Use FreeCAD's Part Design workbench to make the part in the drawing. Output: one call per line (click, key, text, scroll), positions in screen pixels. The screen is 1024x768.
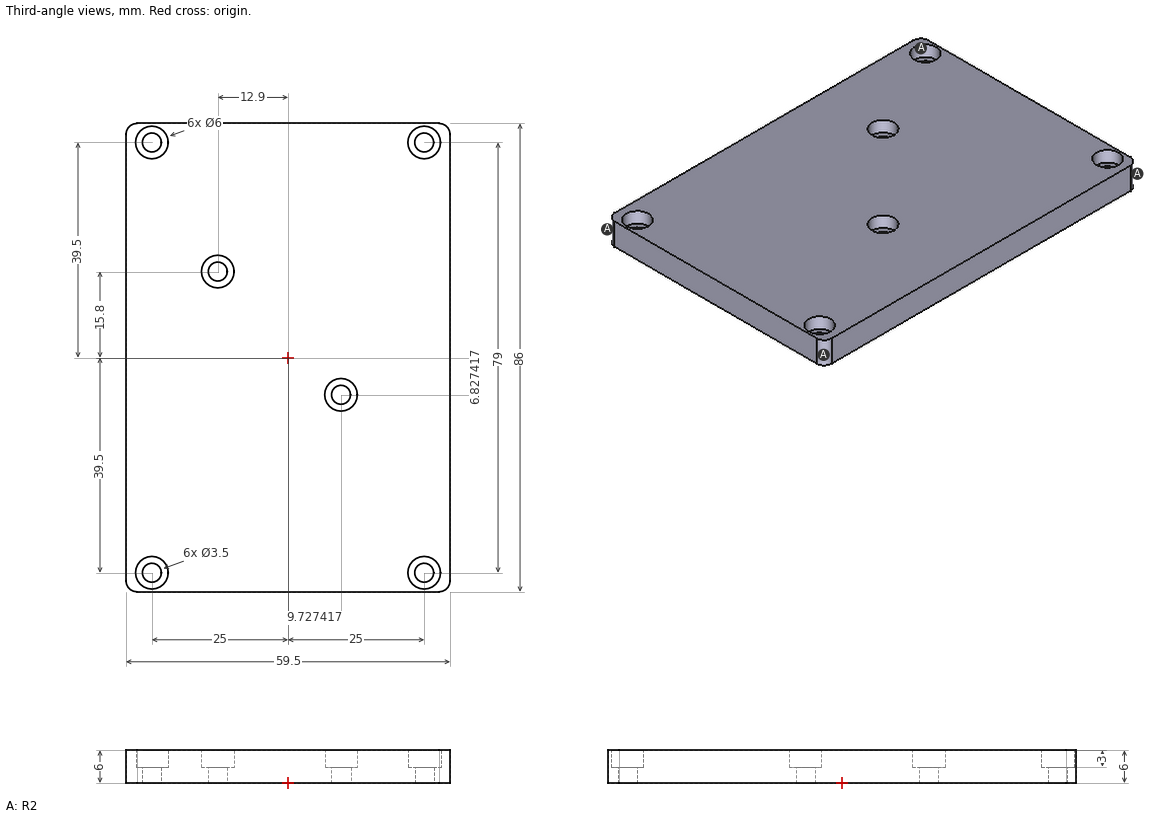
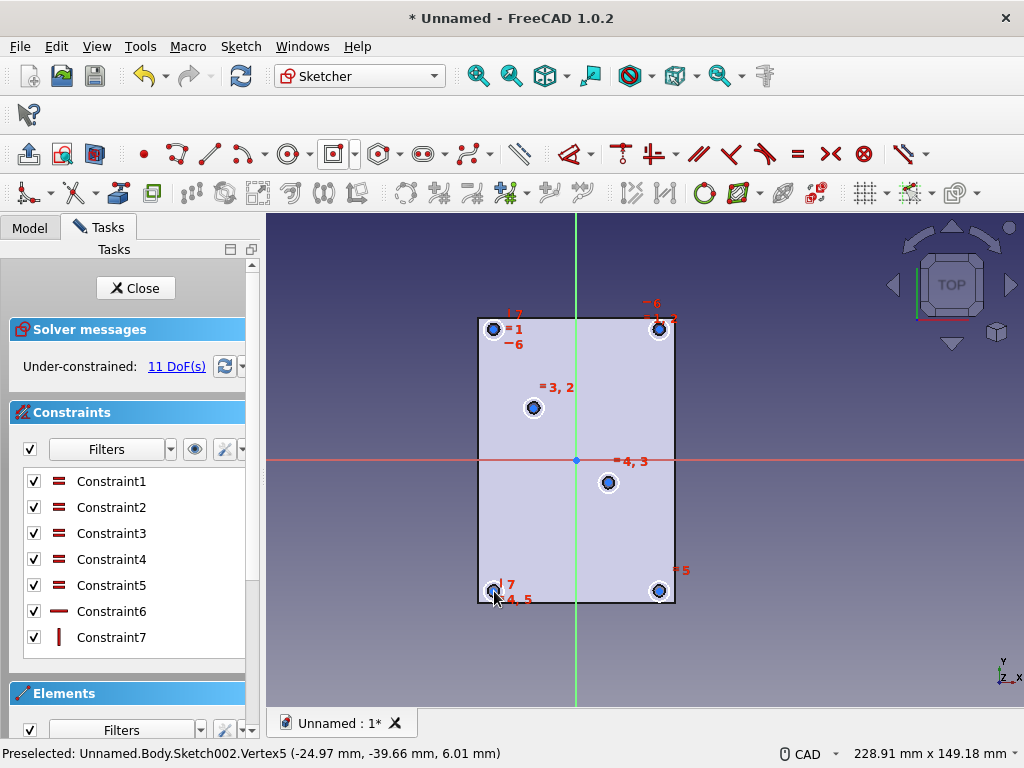
click(659, 330)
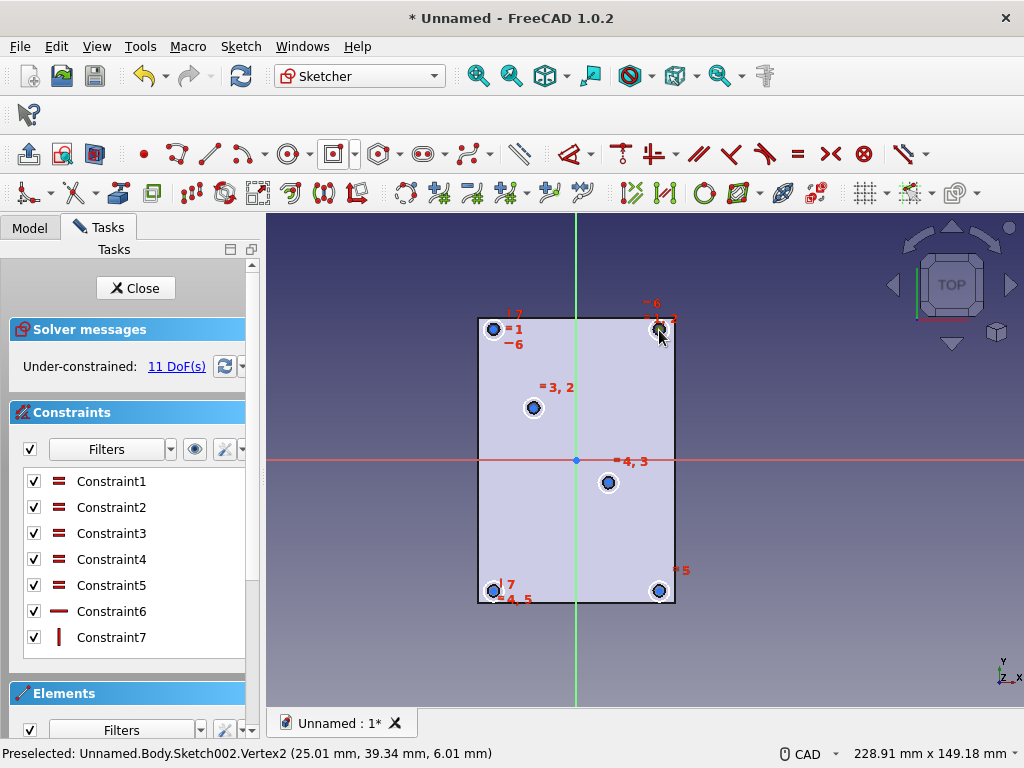
click(659, 591)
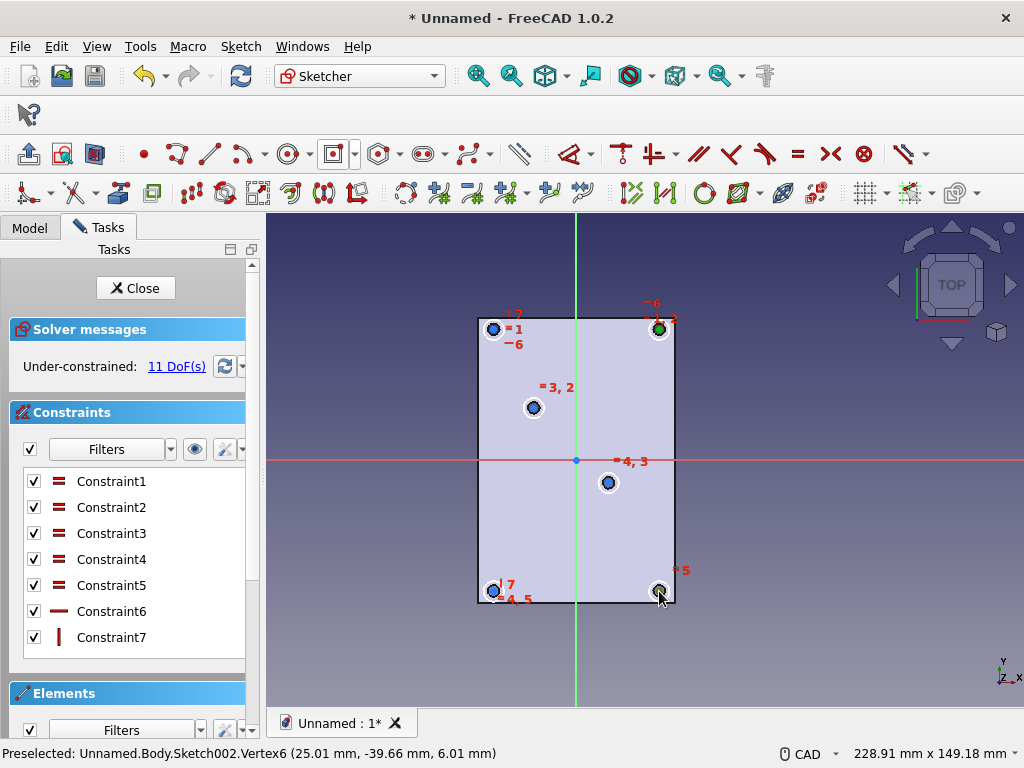
key(v)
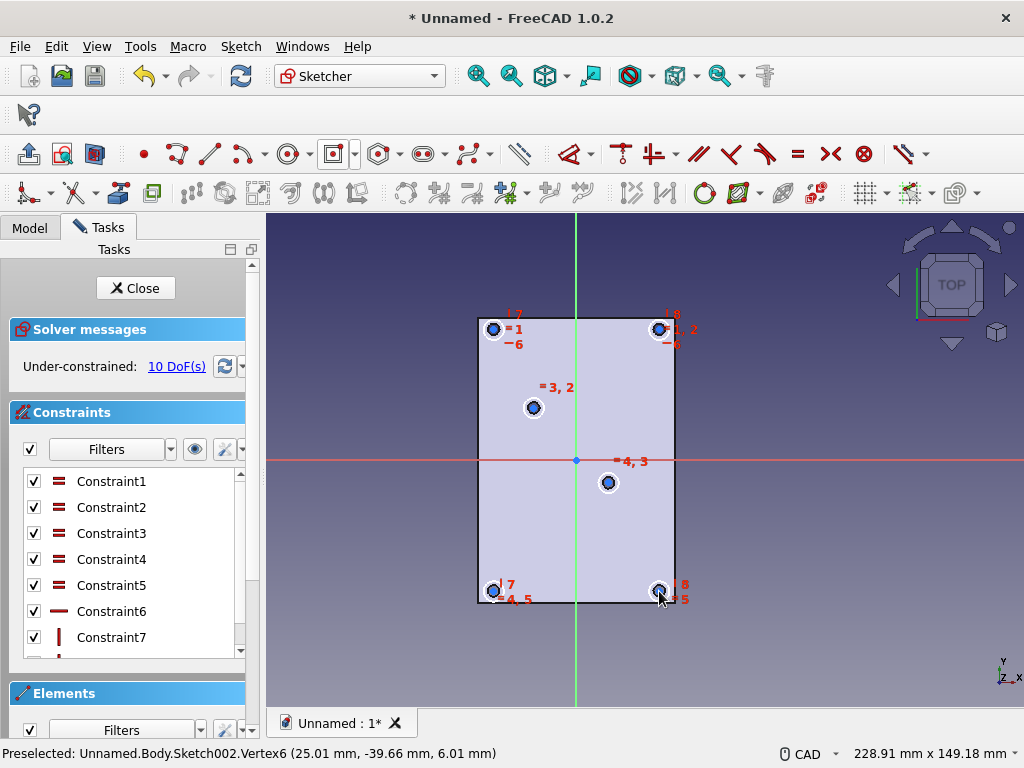
click(494, 591)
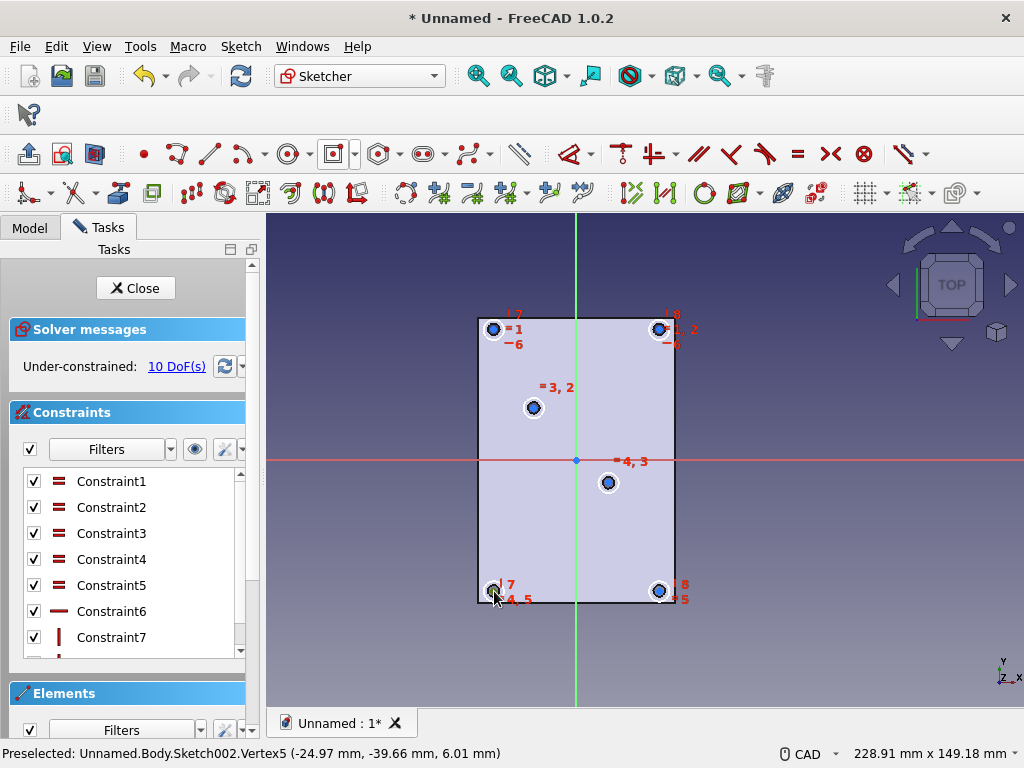
click(659, 591)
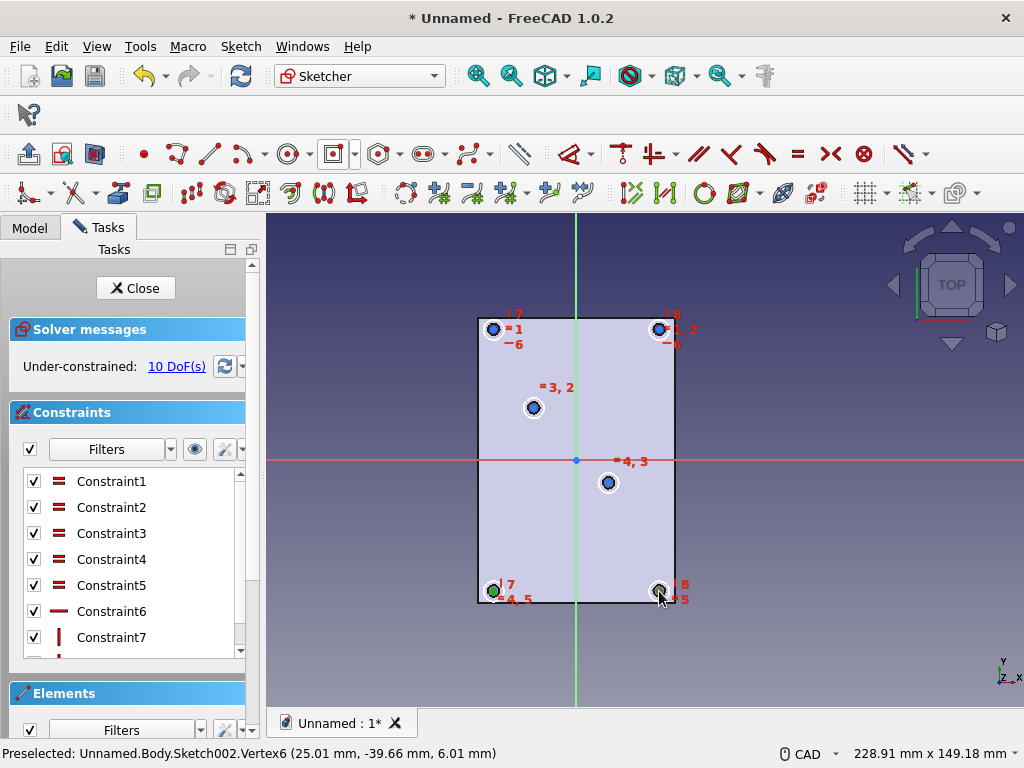
key(h)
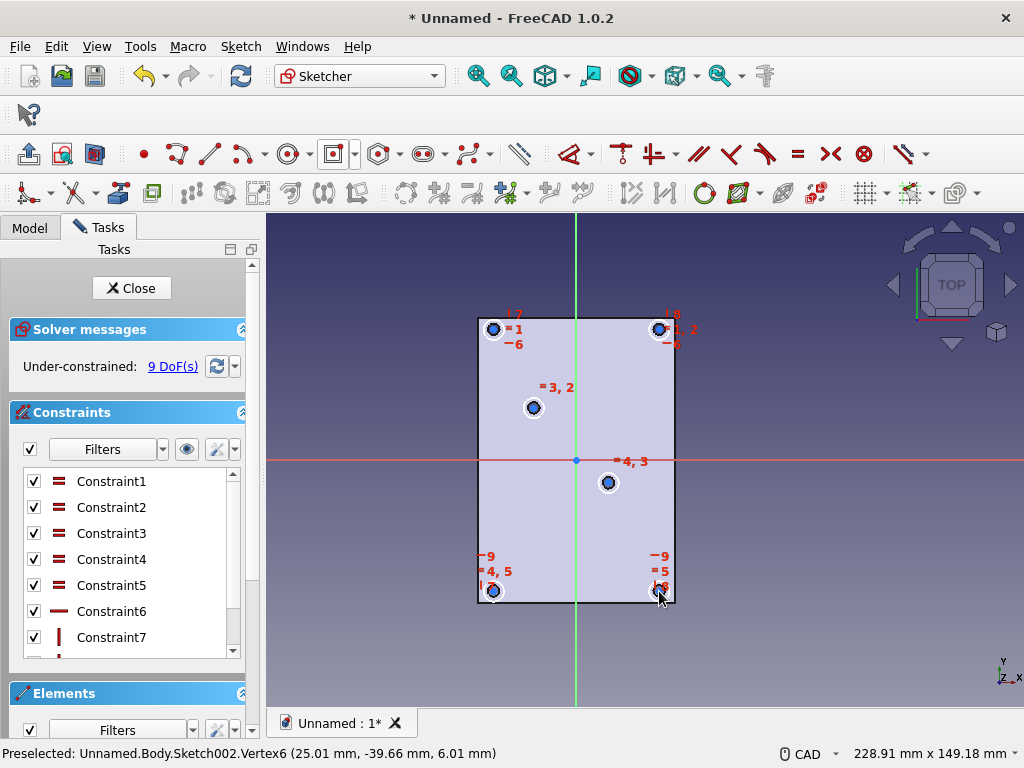
click(568, 154)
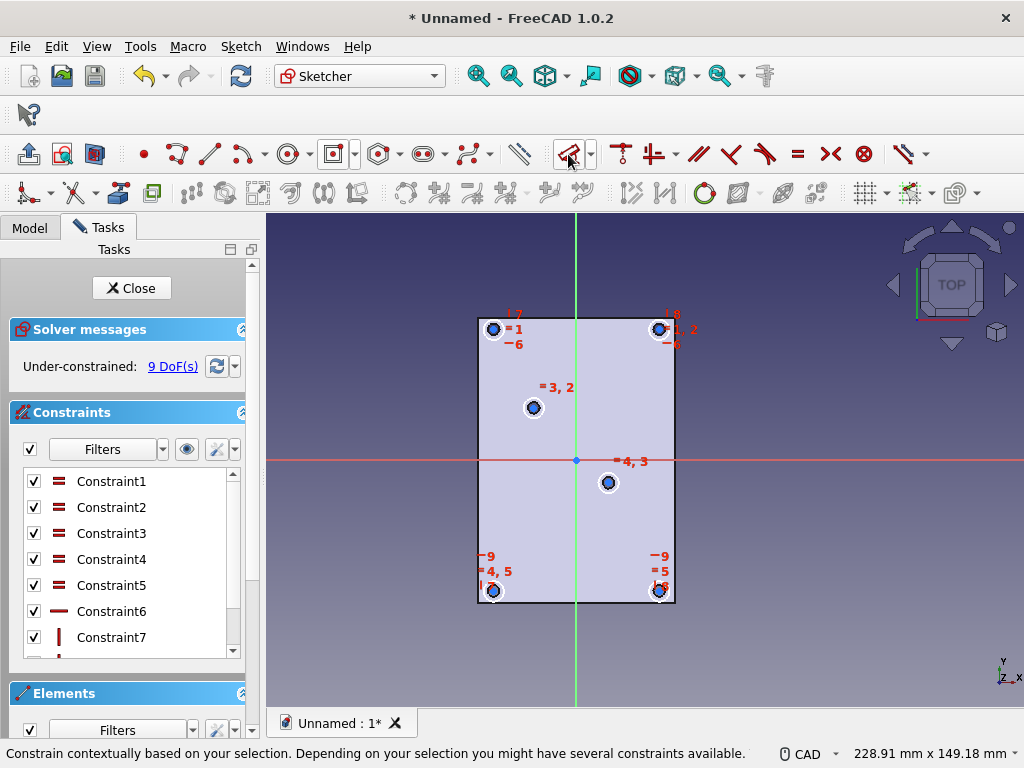
scroll(501, 323, up, 4)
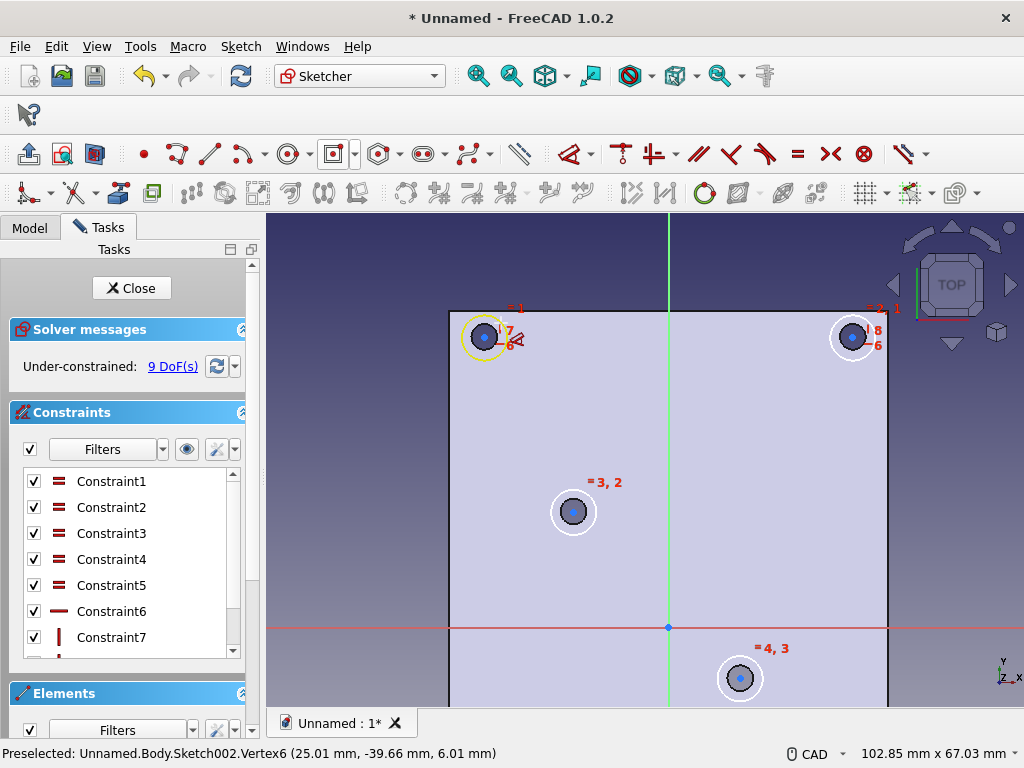
click(501, 322)
click(524, 300)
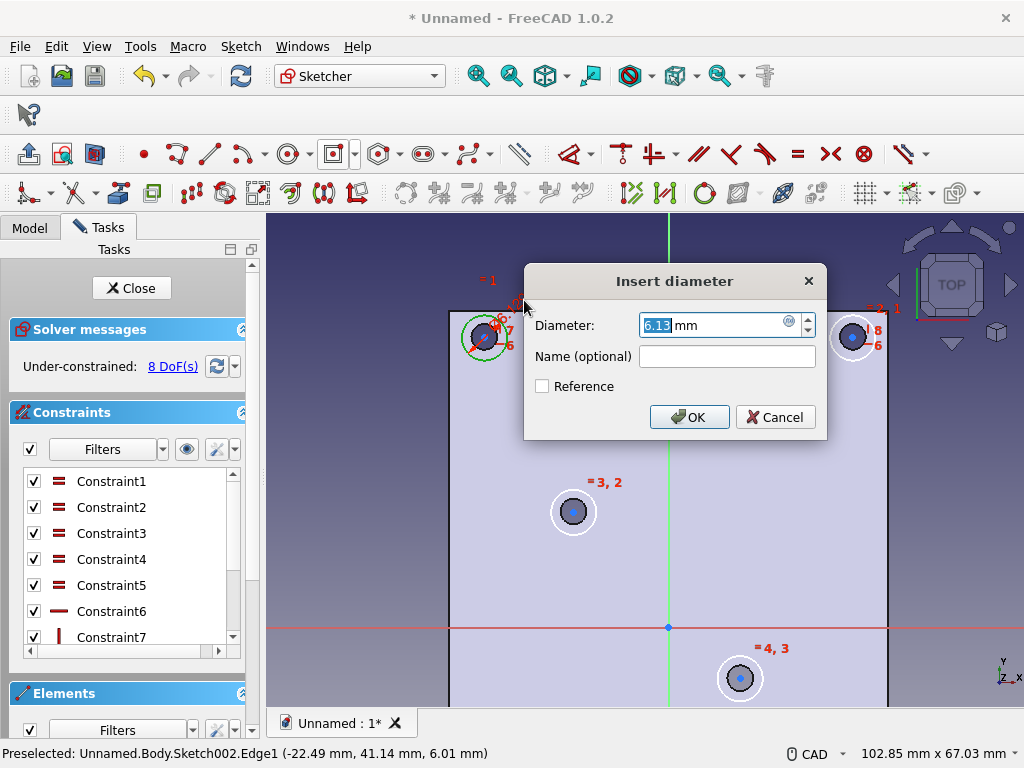
text(6)
key(Return)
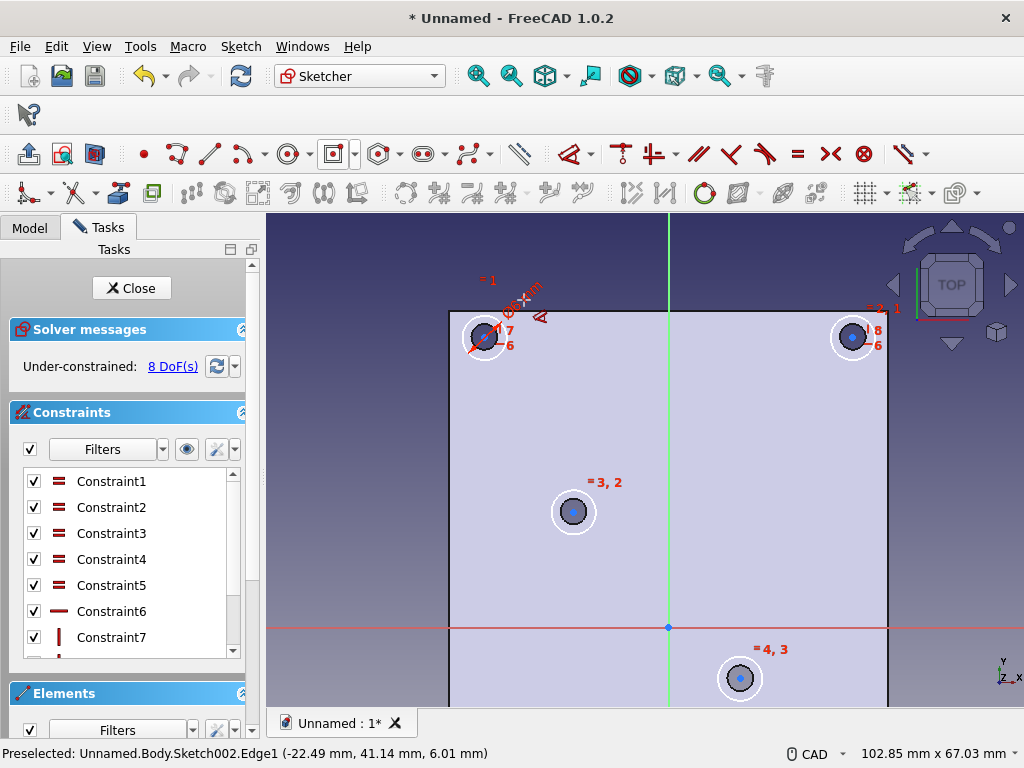
click(485, 338)
click(619, 304)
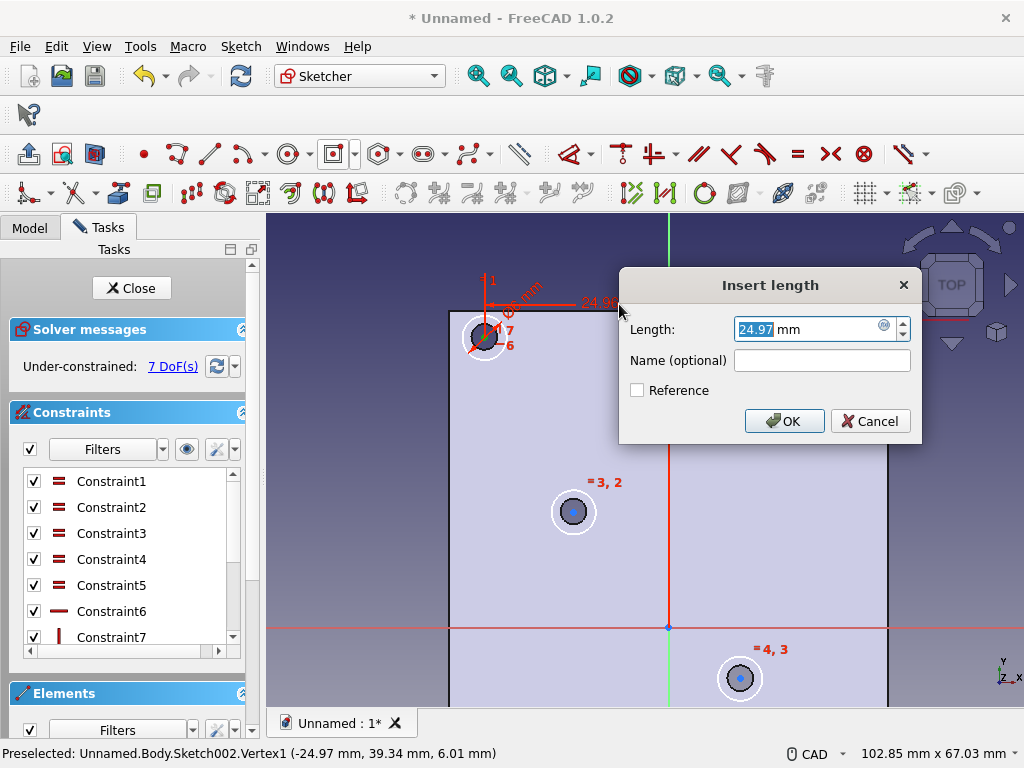
text(25)
key(Return)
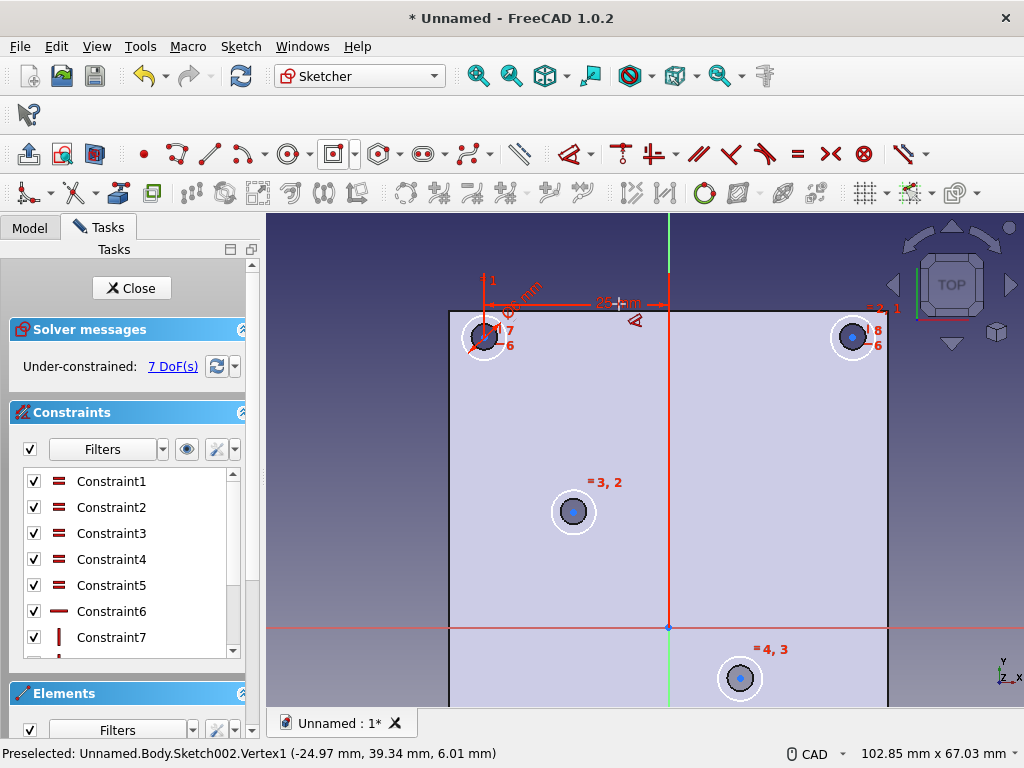
click(853, 338)
click(761, 304)